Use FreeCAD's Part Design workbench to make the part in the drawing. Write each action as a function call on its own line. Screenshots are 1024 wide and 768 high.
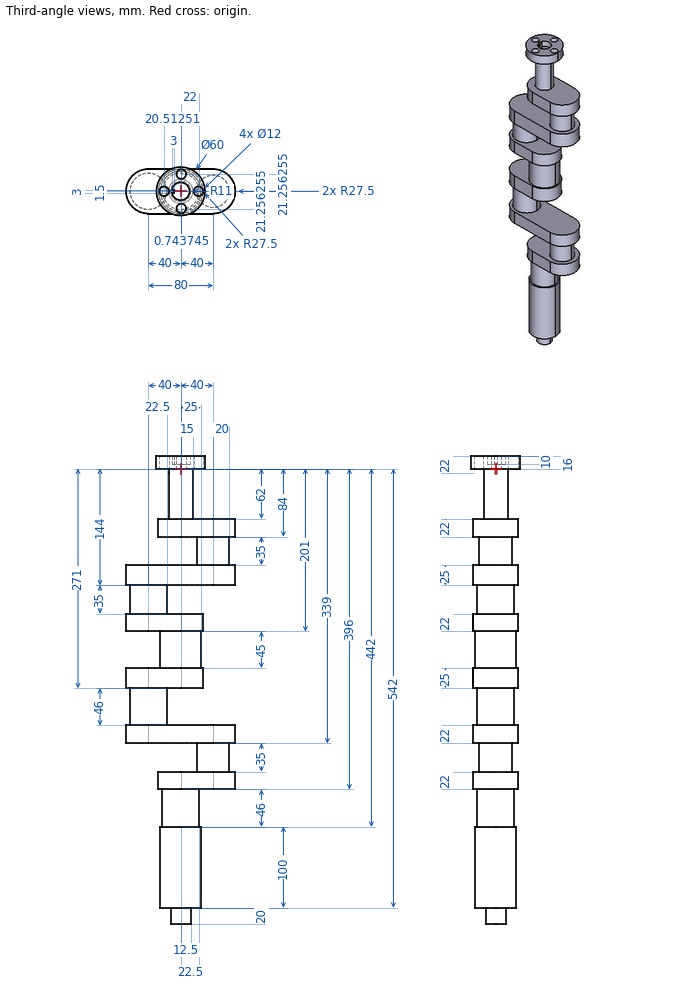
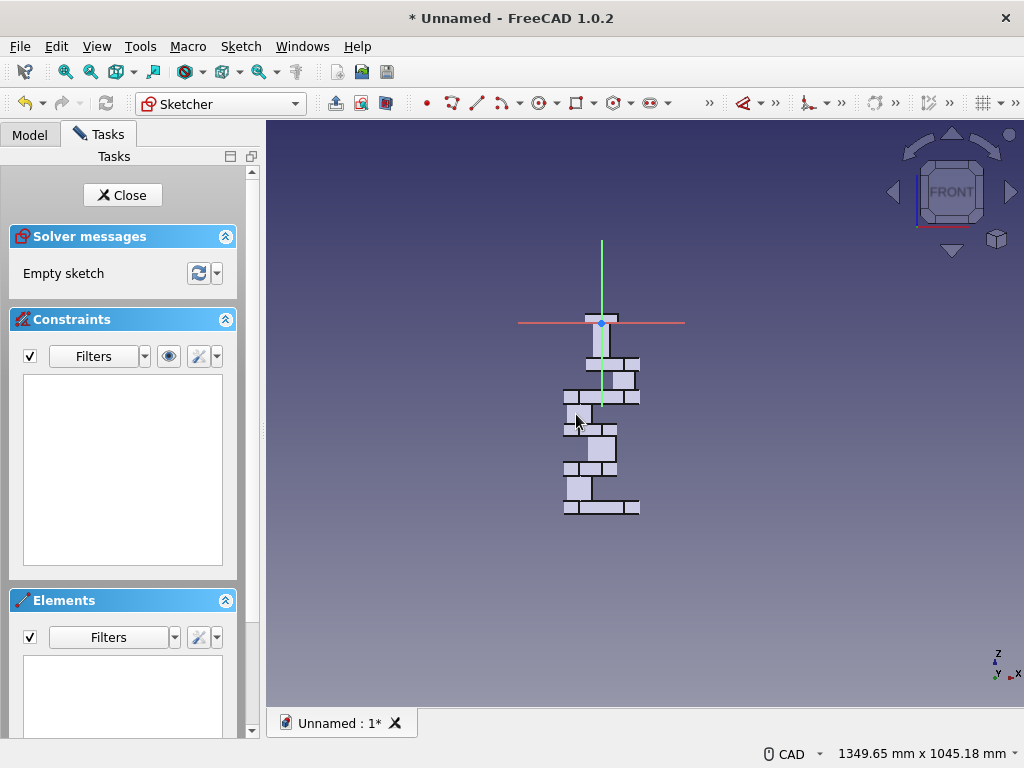
scroll(634, 537, up, 13)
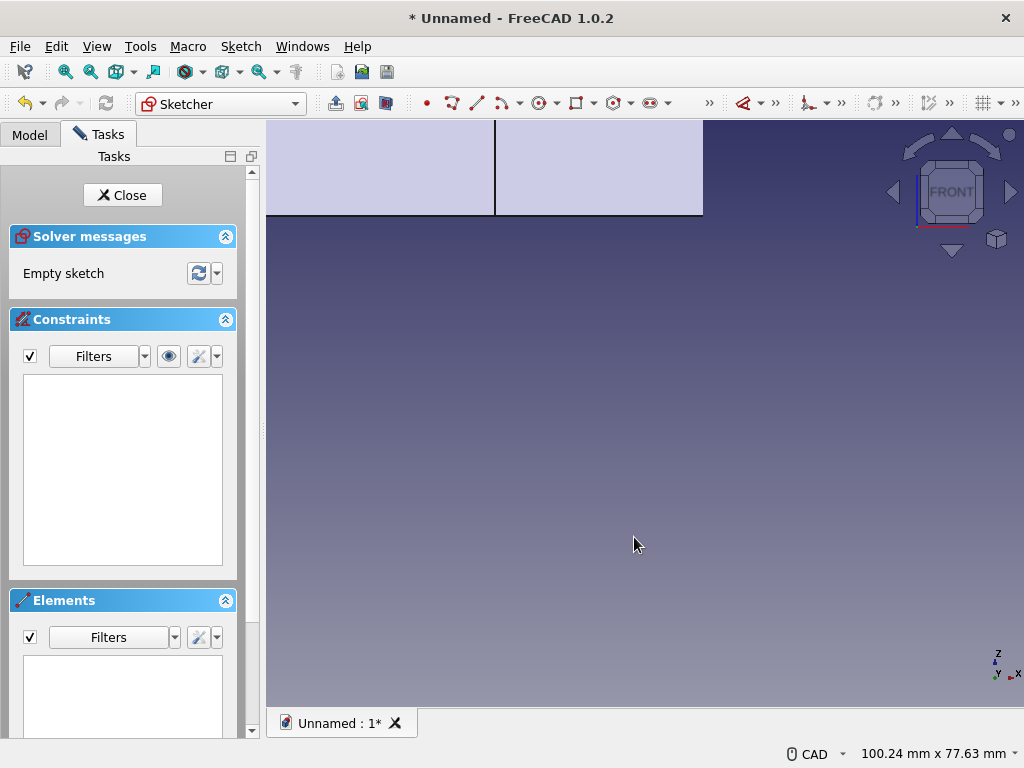
key(g)
key(r)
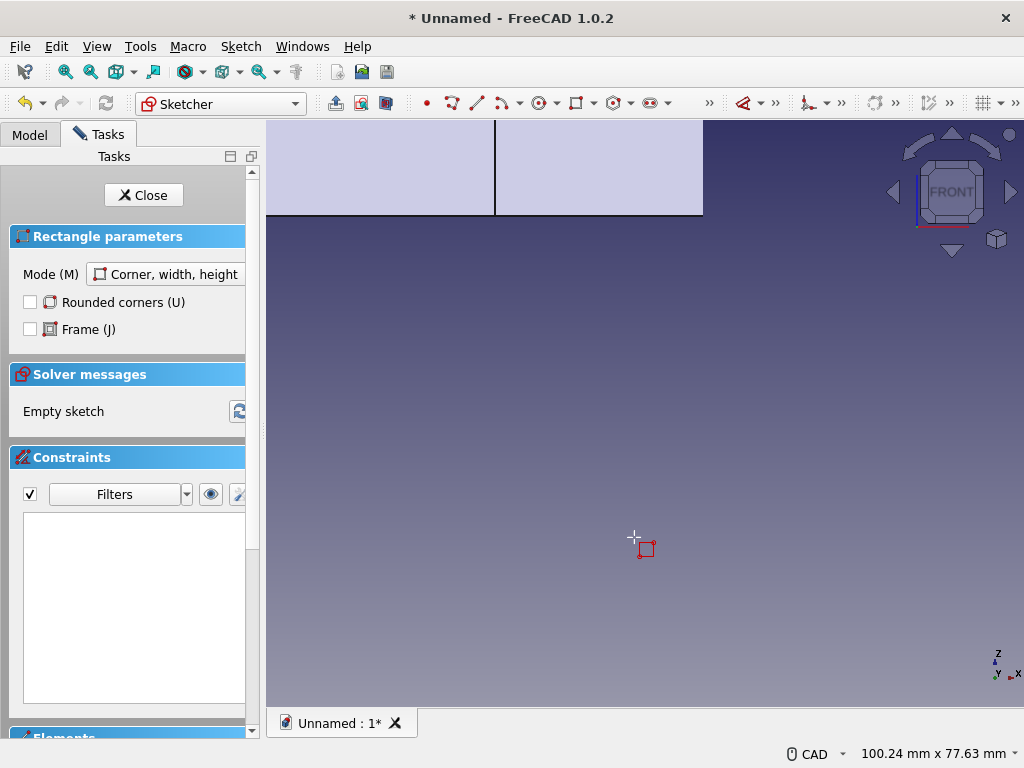
click(495, 216)
move(646, 481)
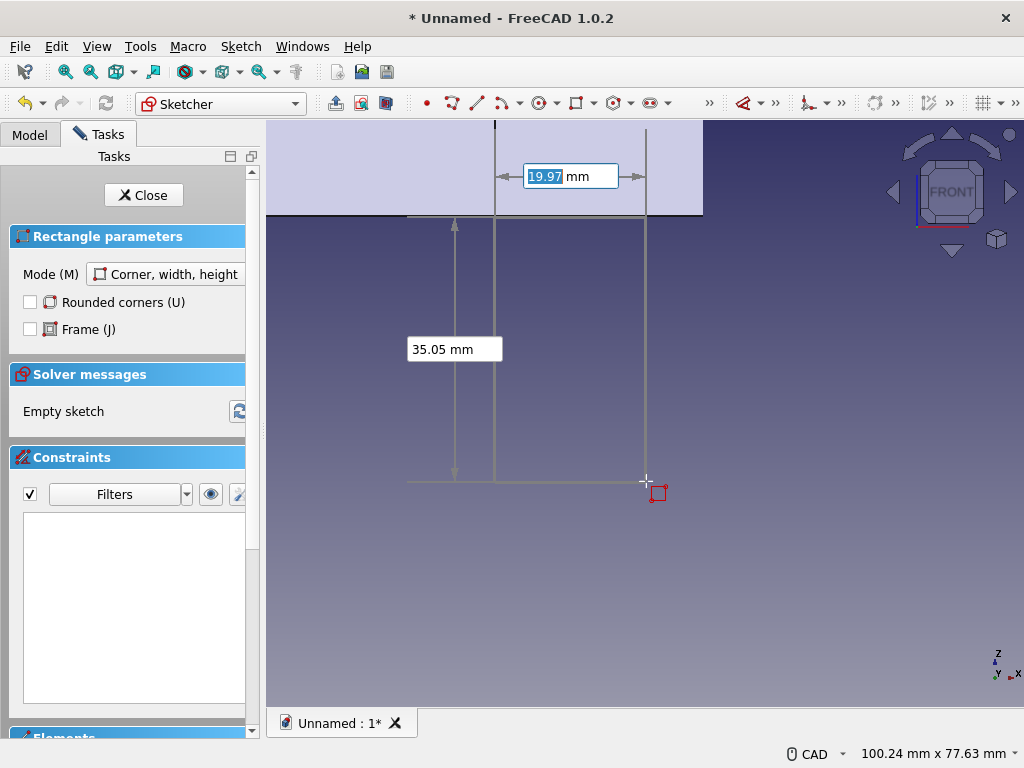
text(20)
key(Tab)
text(35)
key(Return)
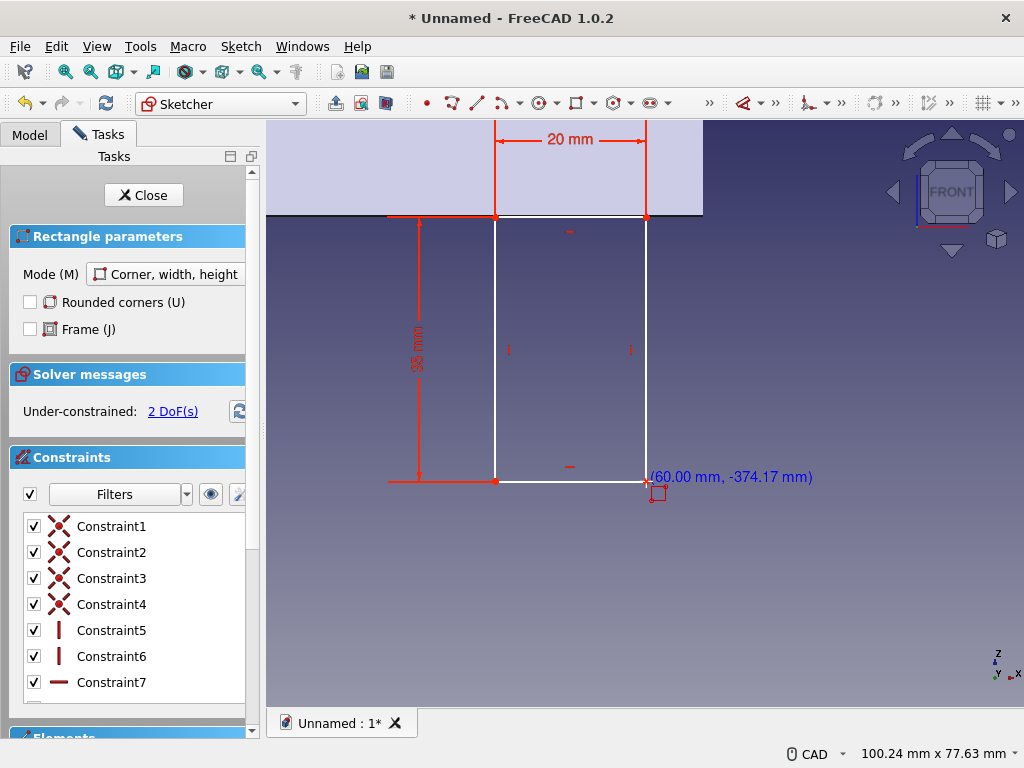
key(g)
key(l)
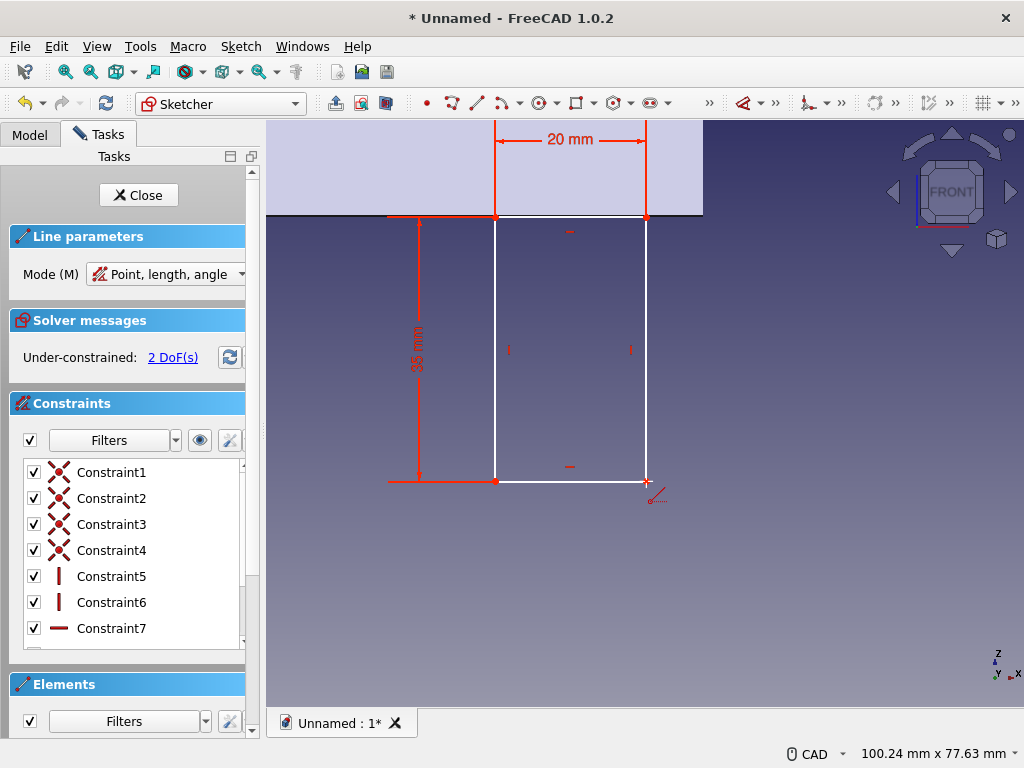
click(495, 507)
click(495, 587)
key(Escape)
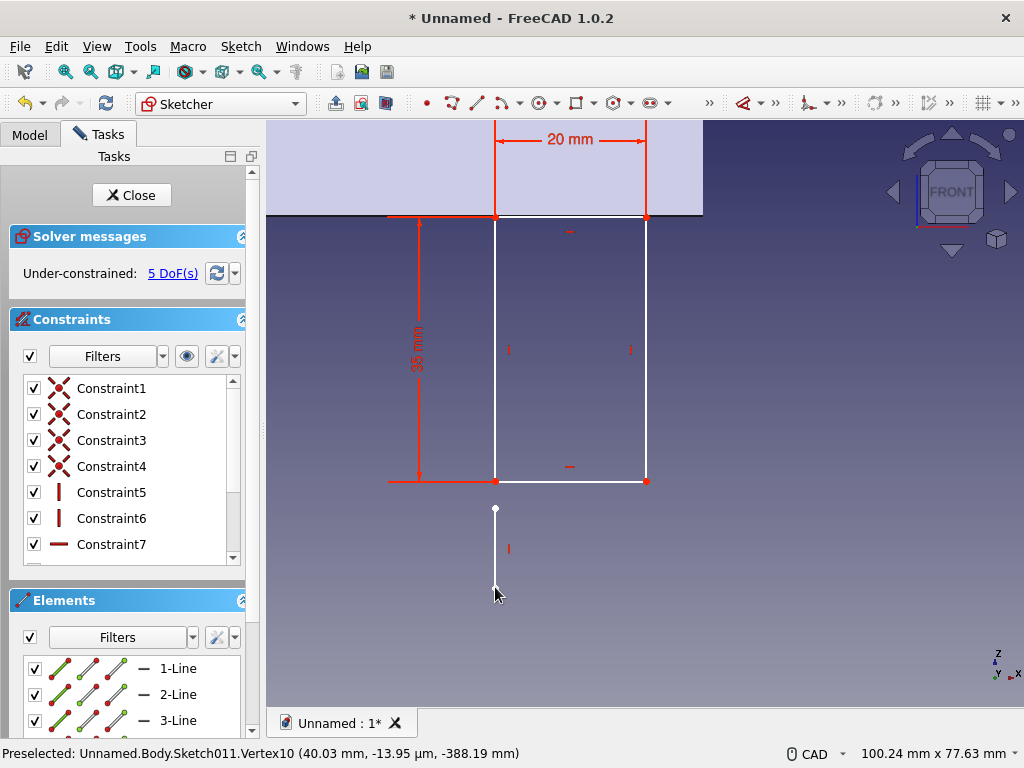
click(495, 532)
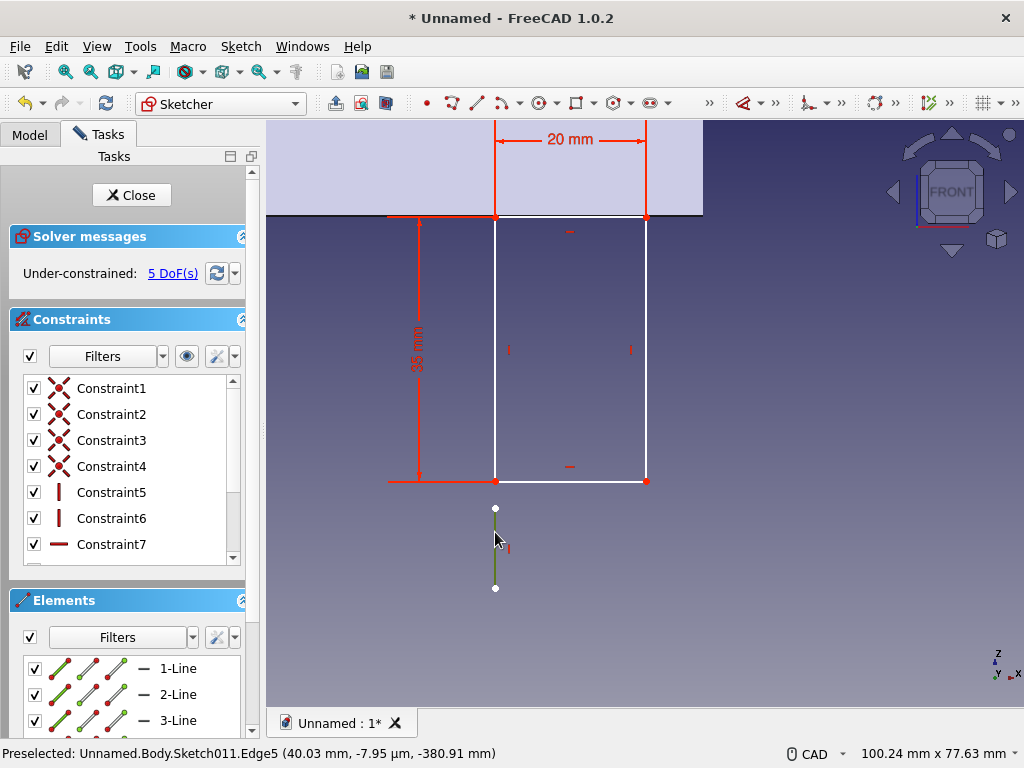
key(g)
key(n)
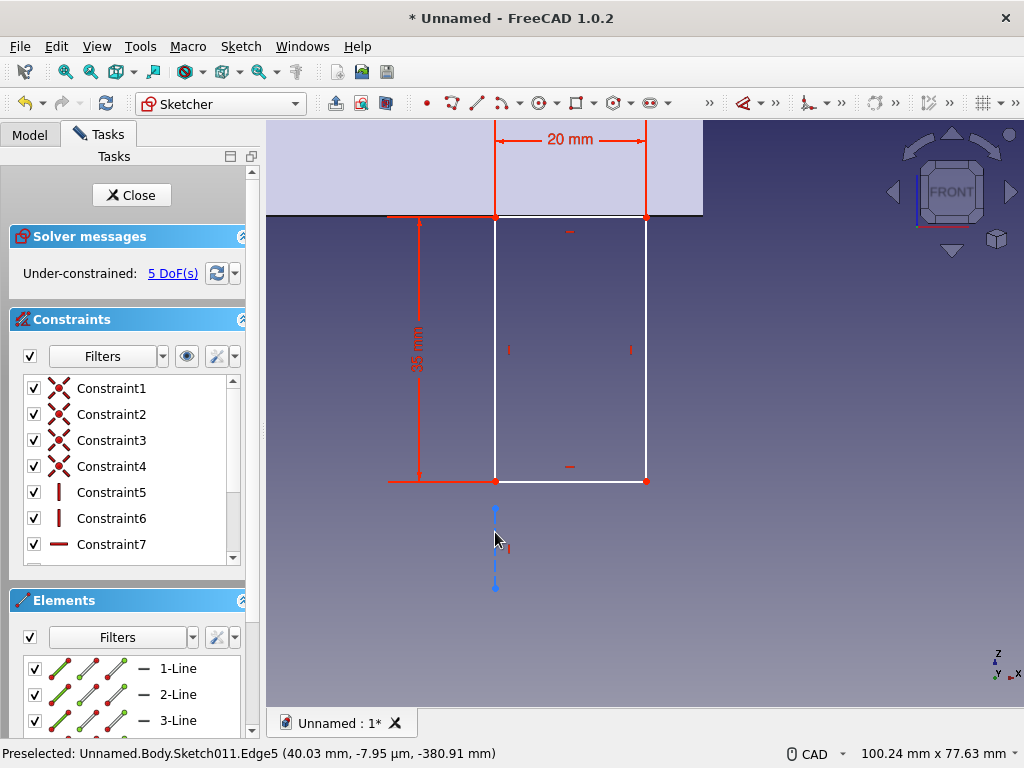
click(742, 104)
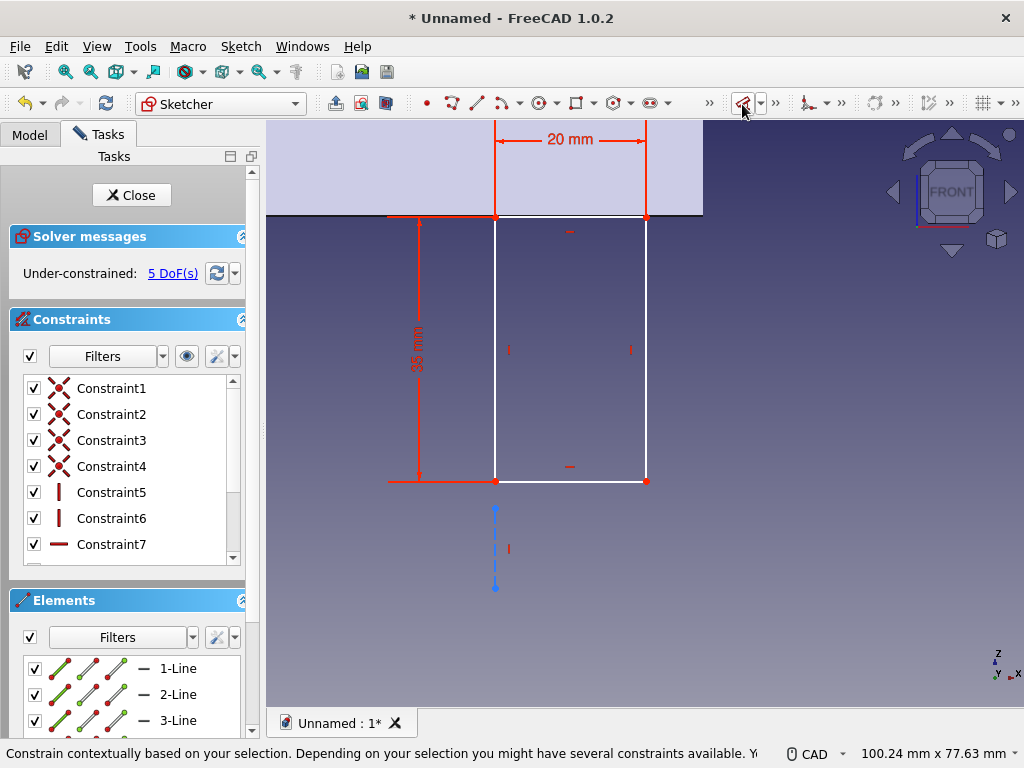
click(495, 217)
click(395, 251)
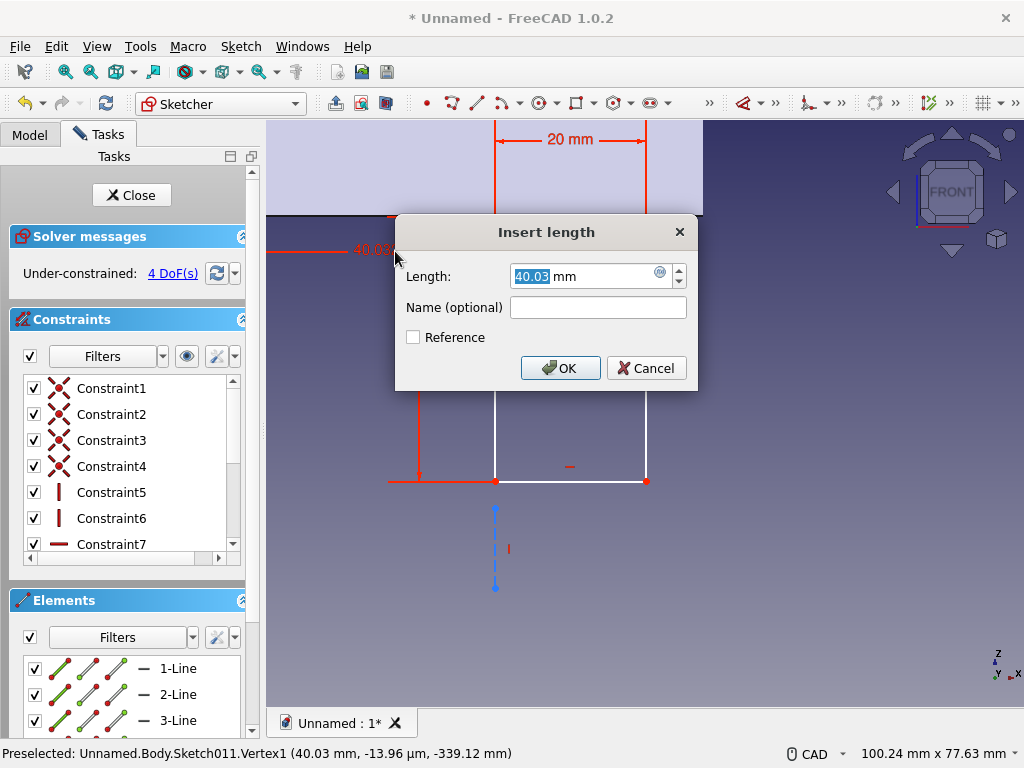
text(40)
key(Return)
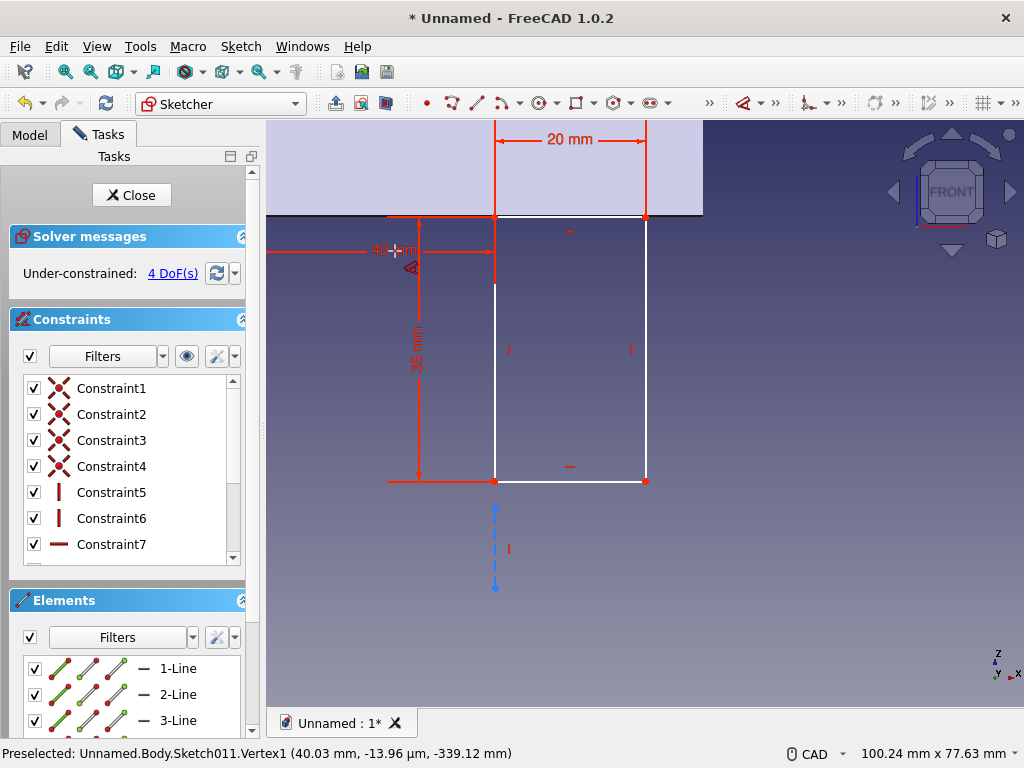
click(495, 508)
click(395, 542)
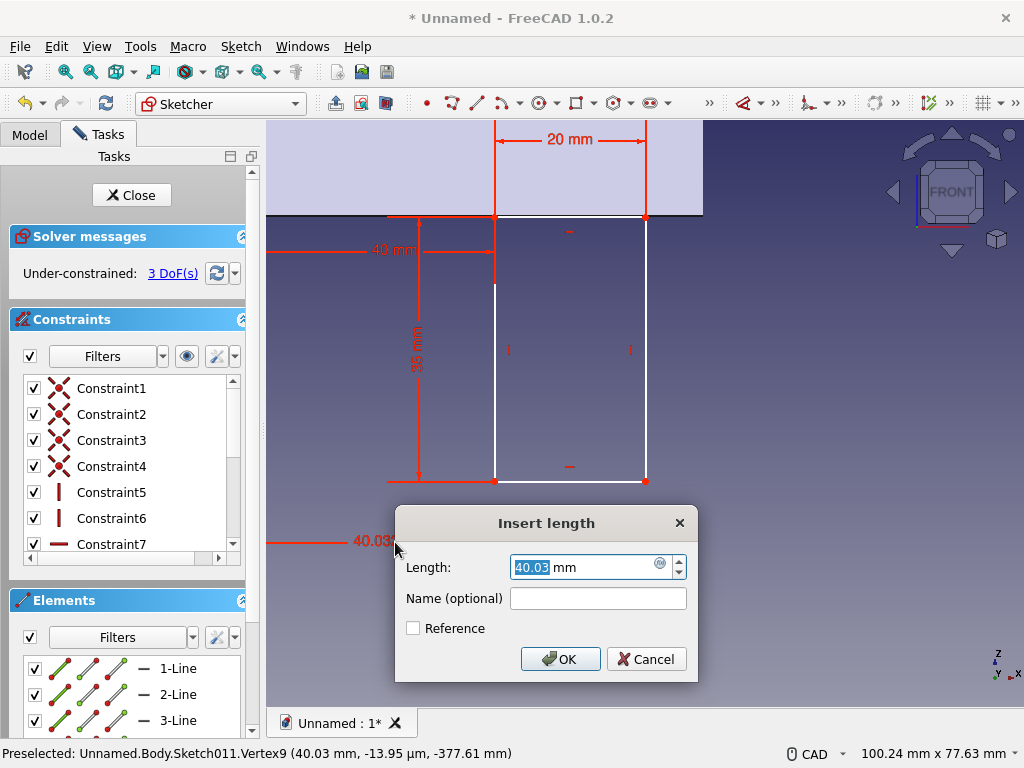
text(40)
key(Return)